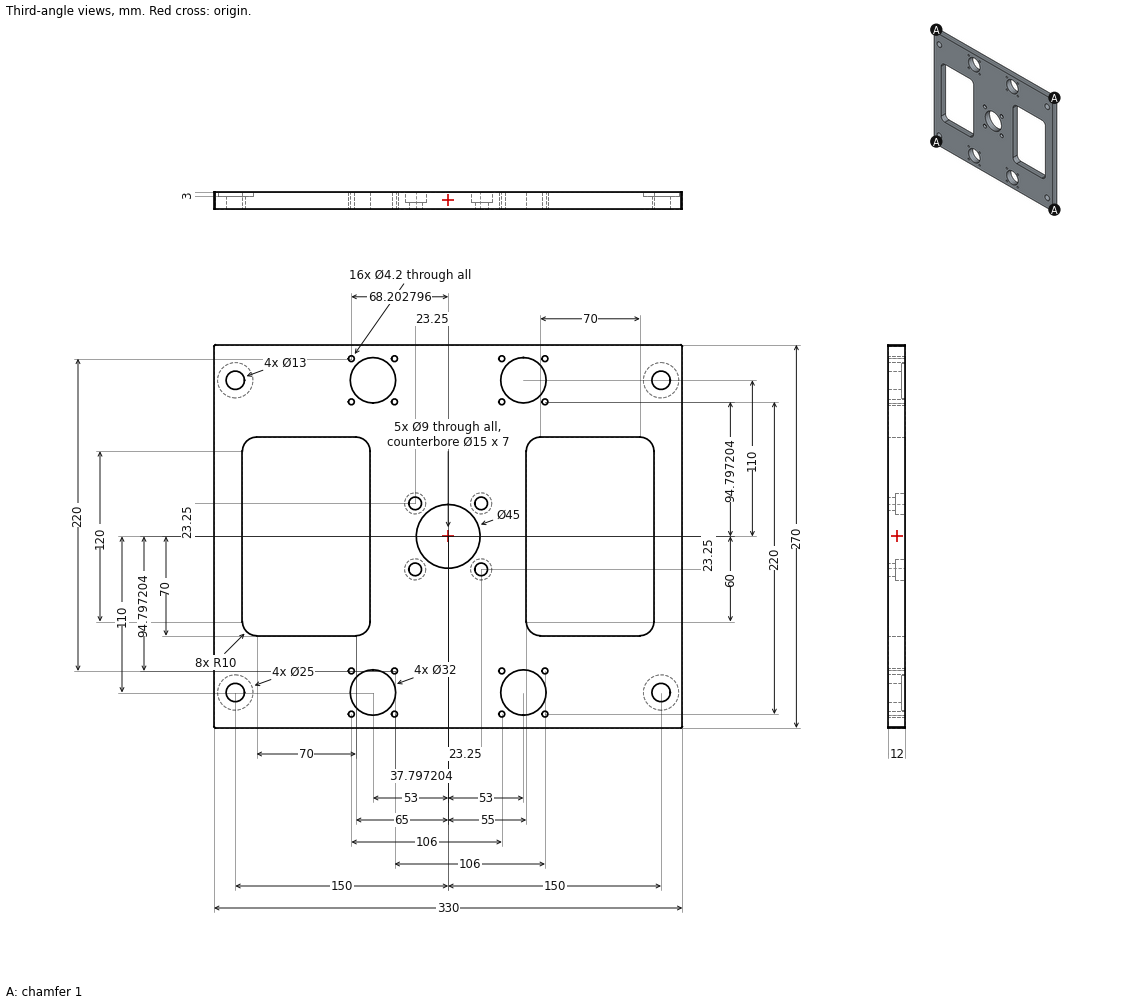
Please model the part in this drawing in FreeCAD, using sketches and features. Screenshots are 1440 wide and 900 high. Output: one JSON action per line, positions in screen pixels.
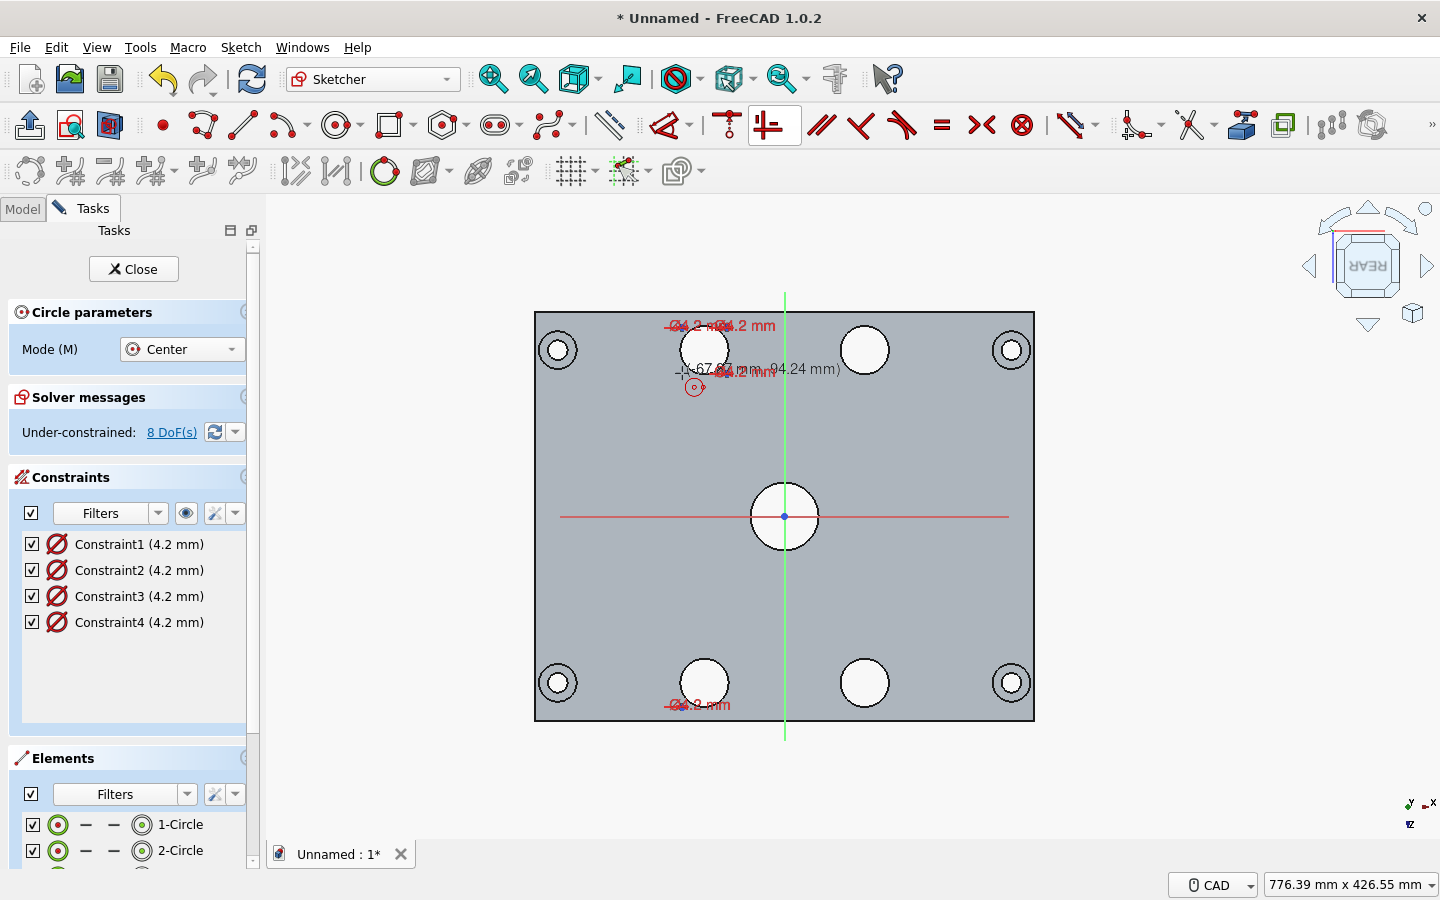
{"action": "left_click", "coordinate": [682, 373]}
{"action": "mouse_move", "coordinate": [684, 371]}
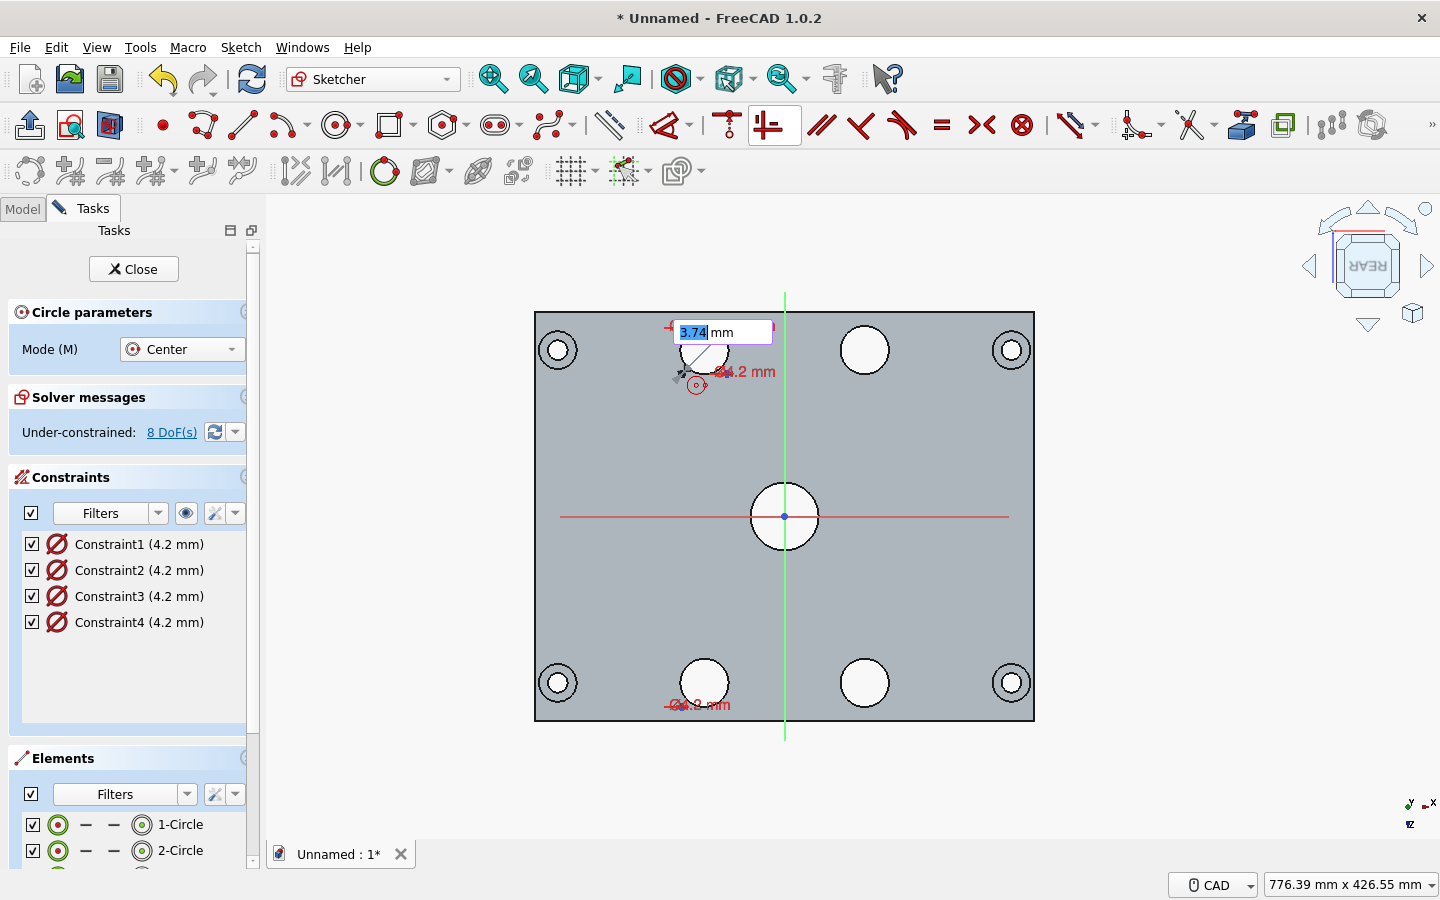
{"action": "type", "text": "4.2"}
{"action": "key", "text": "Return"}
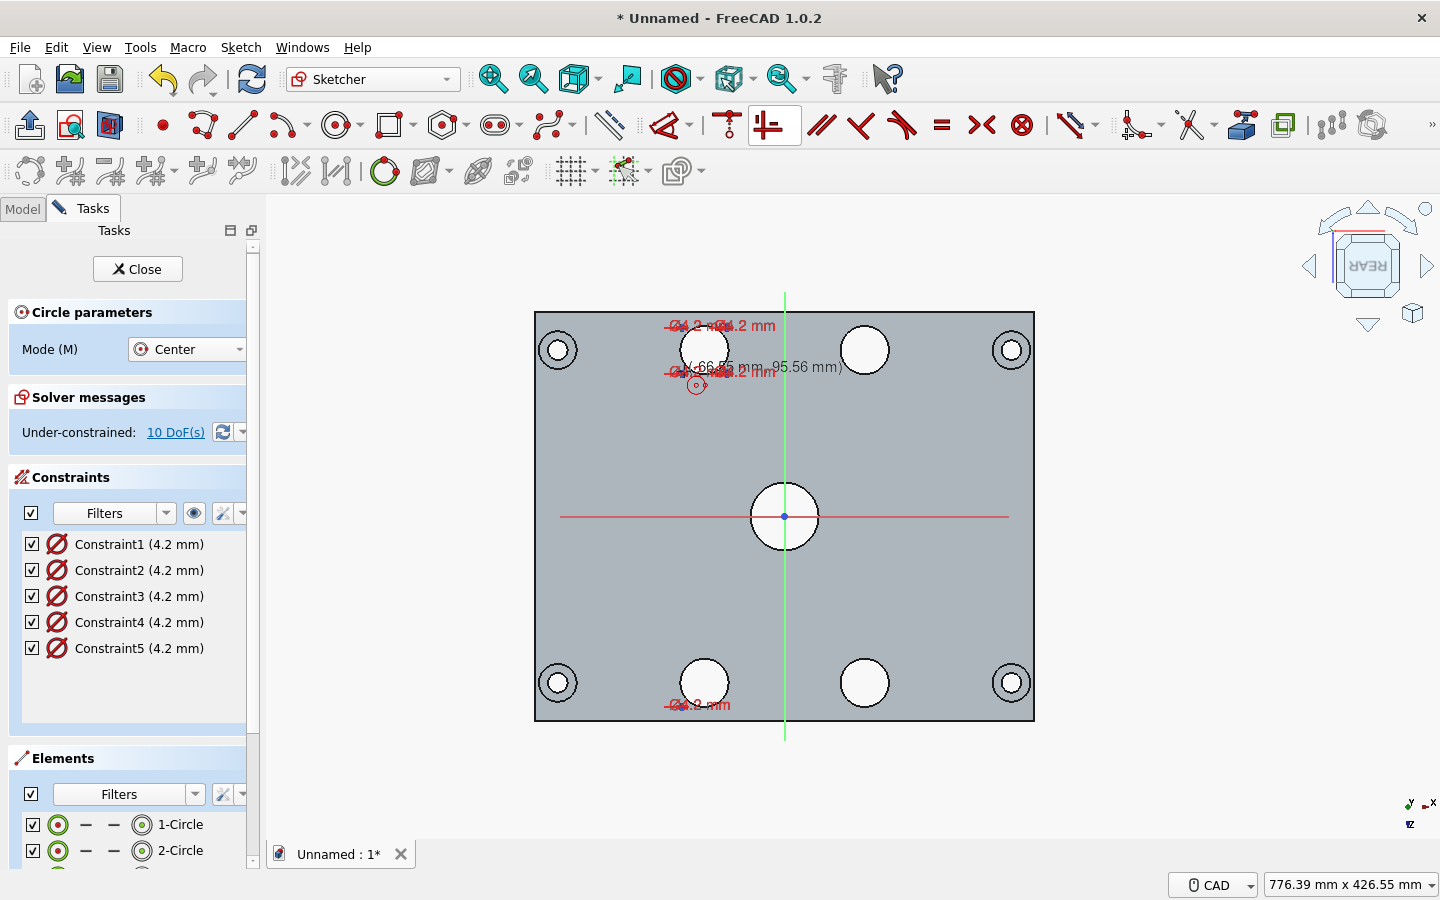
{"action": "scroll", "coordinate": [842, 327], "scroll_direction": "up", "scroll_amount": 10}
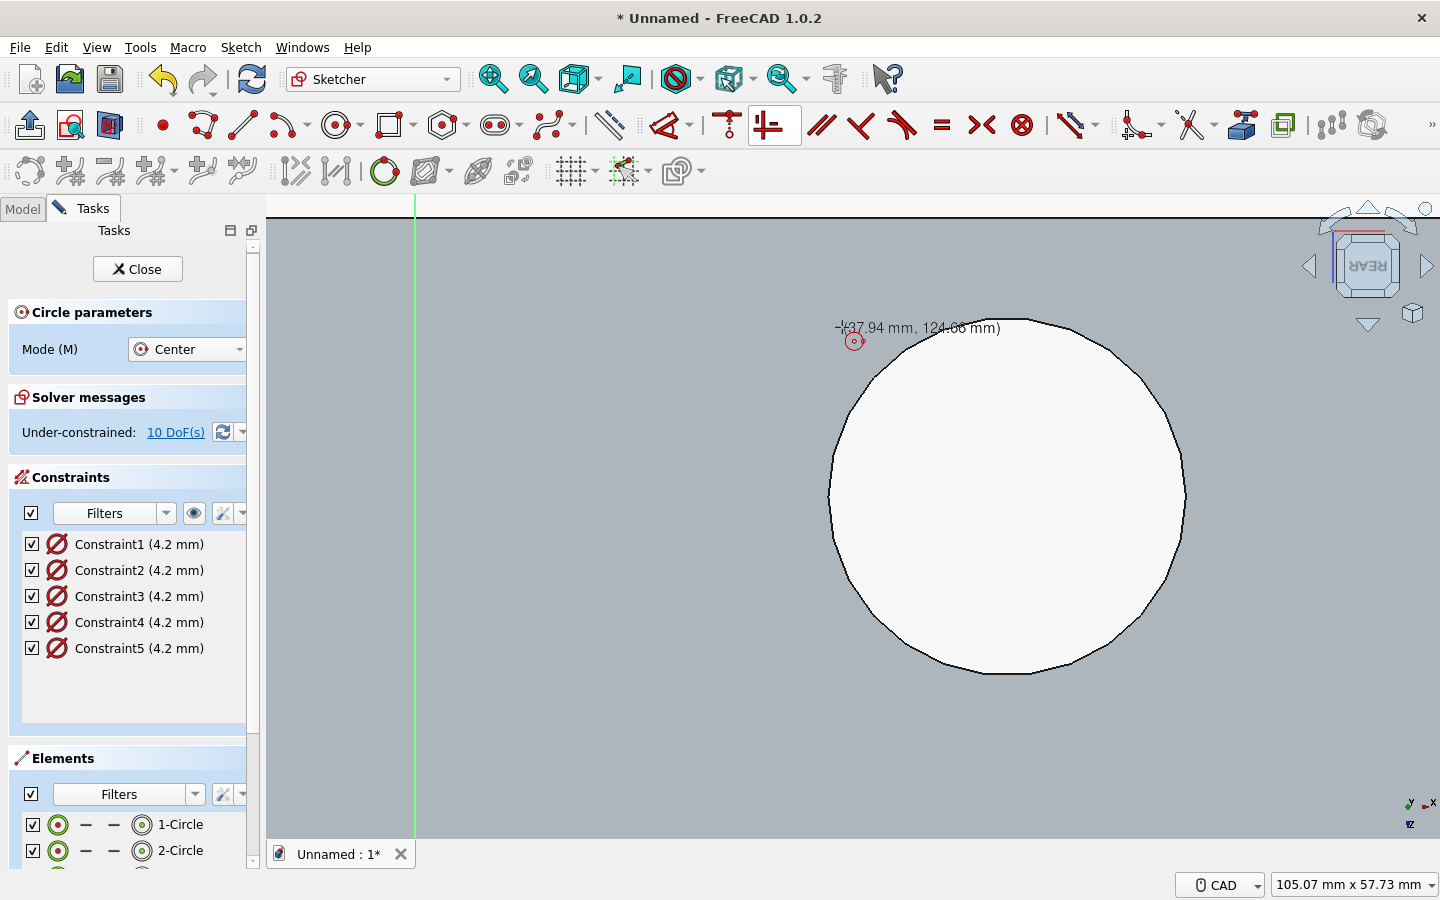
{"action": "scroll", "coordinate": [842, 327], "scroll_direction": "down", "scroll_amount": 10}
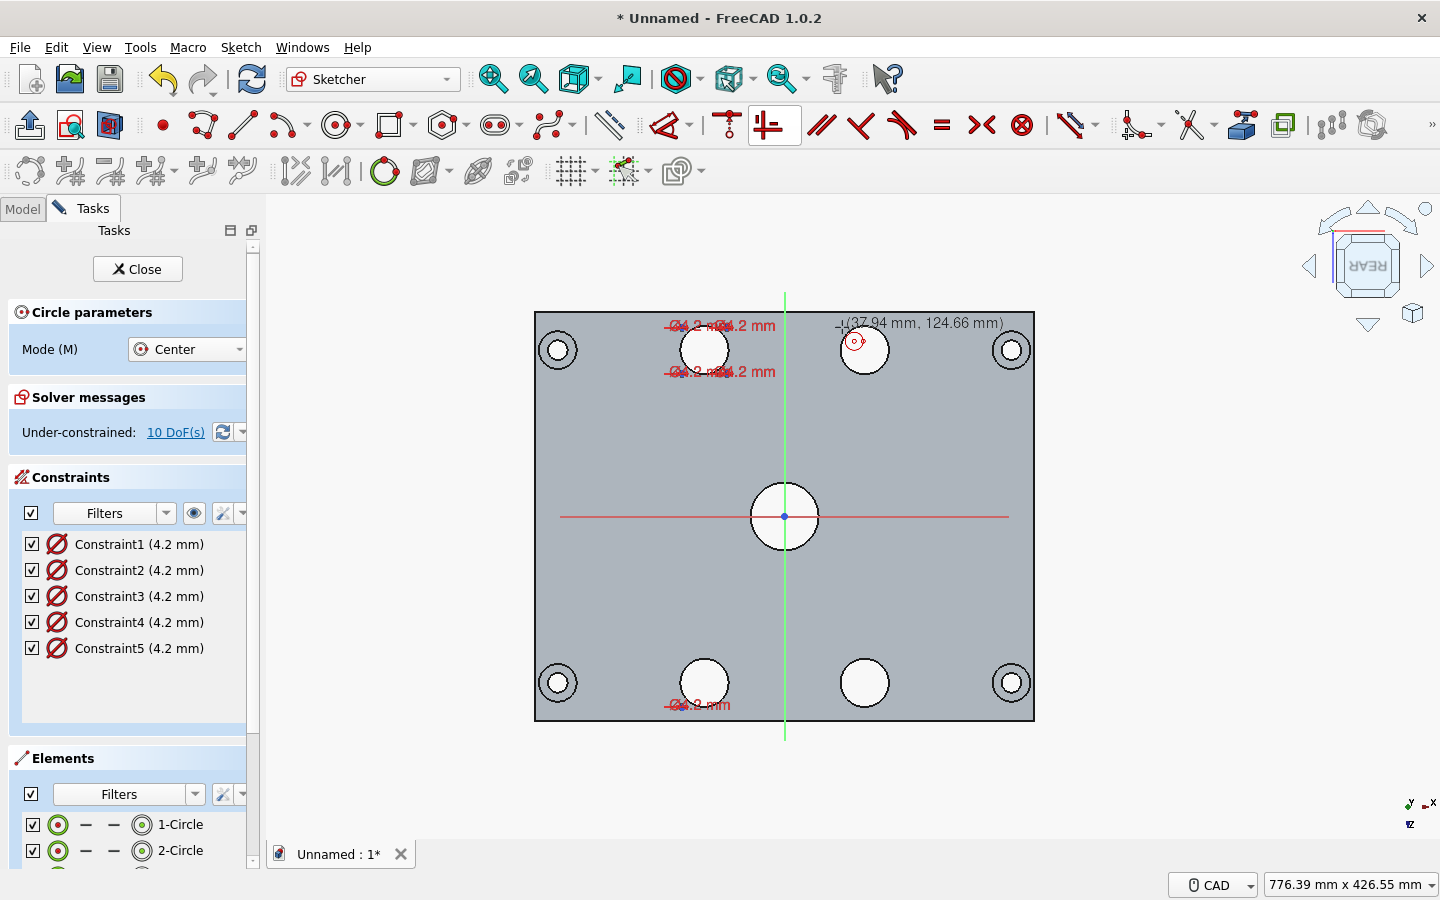
{"action": "left_click", "coordinate": [842, 327]}
{"action": "mouse_move", "coordinate": [844, 325]}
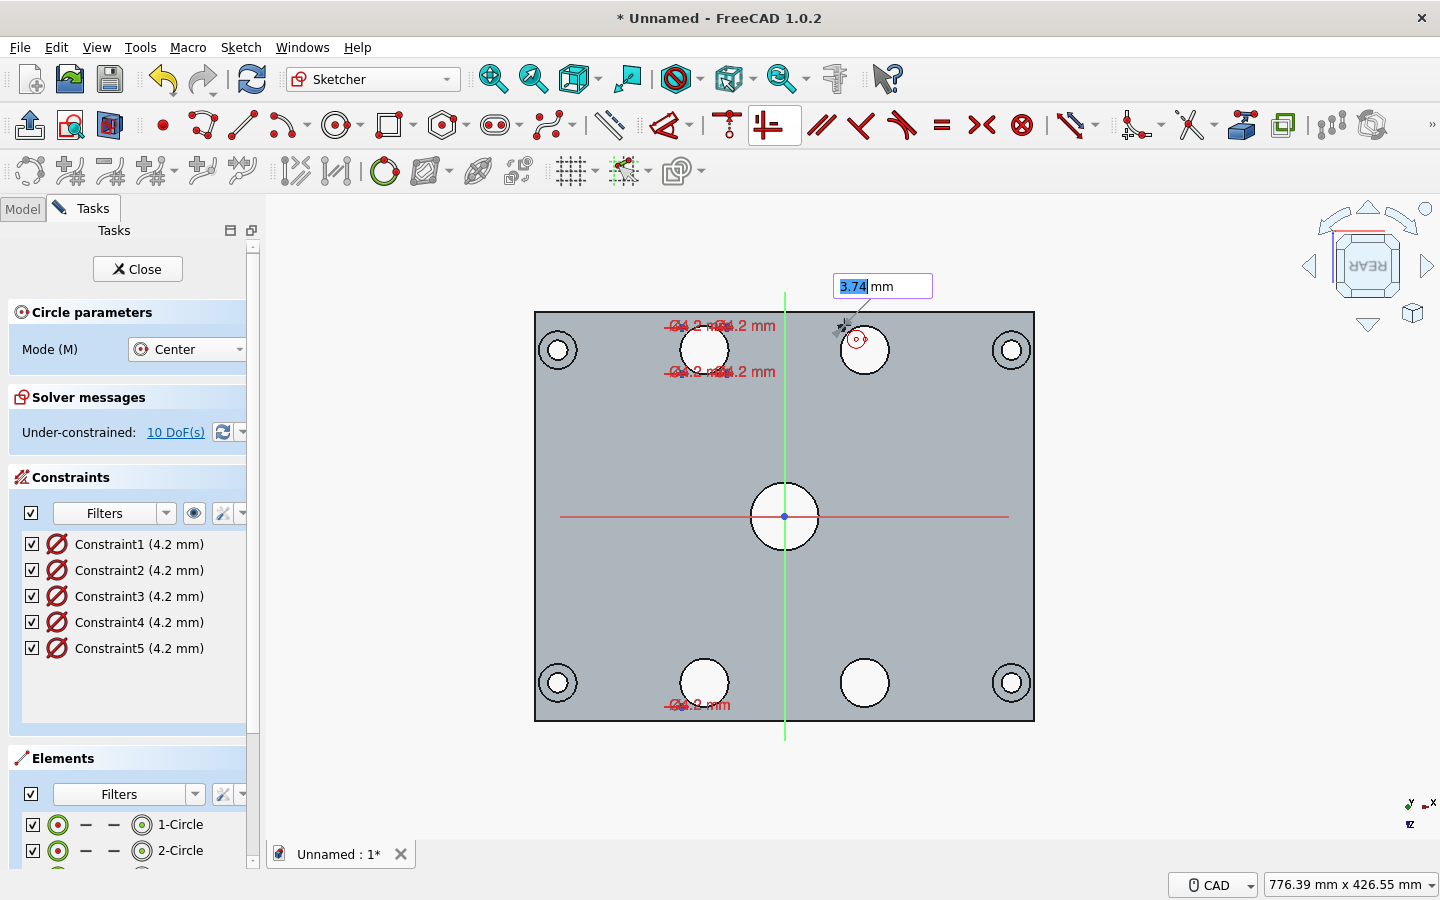
{"action": "type", "text": "4.2"}
{"action": "key", "text": "Return"}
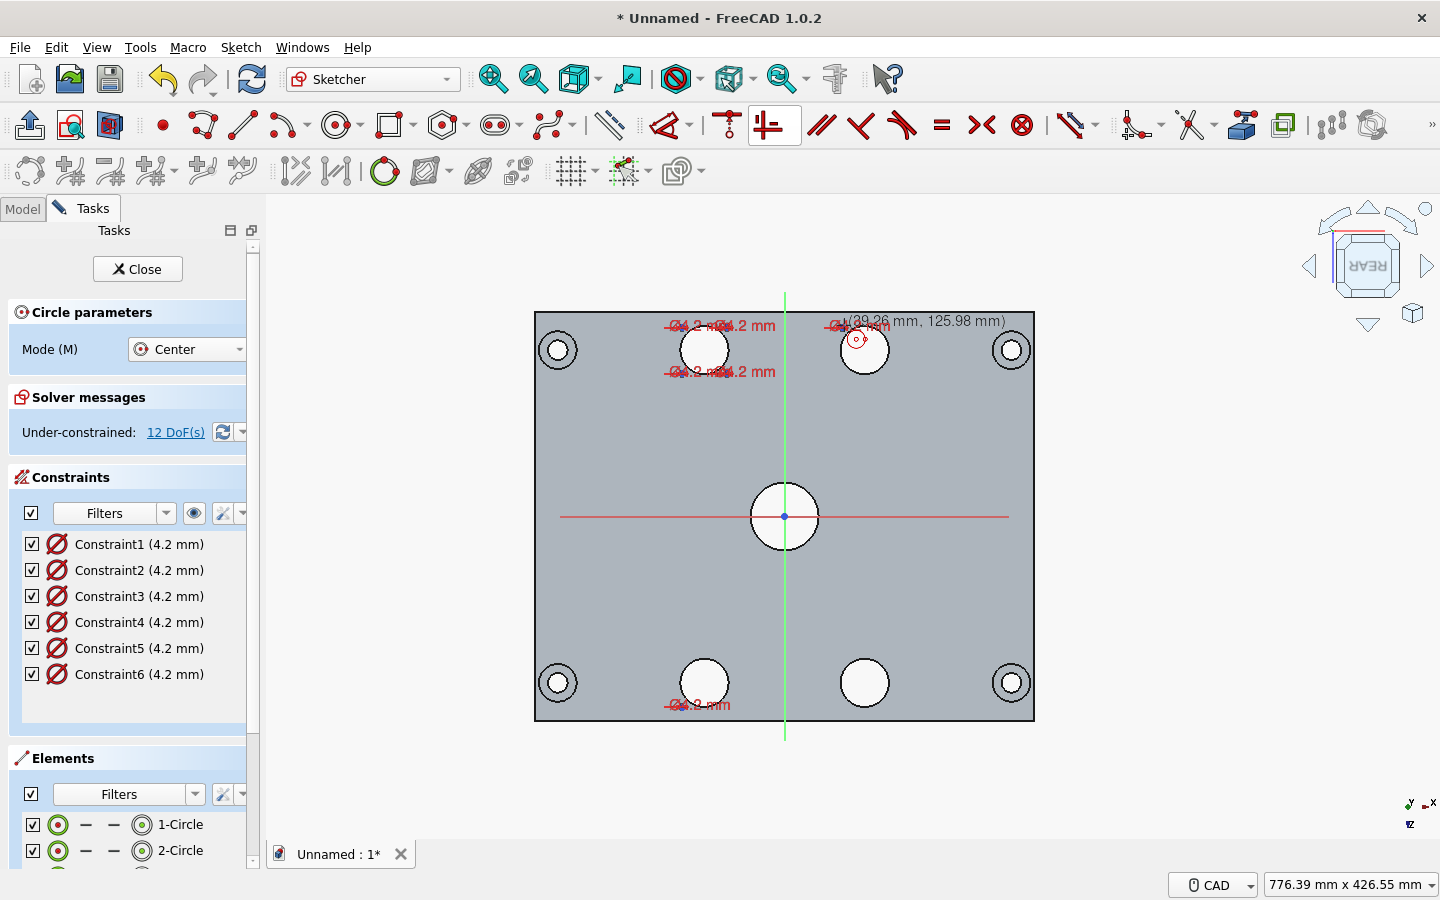
{"action": "scroll", "coordinate": [842, 373], "scroll_direction": "up", "scroll_amount": 10}